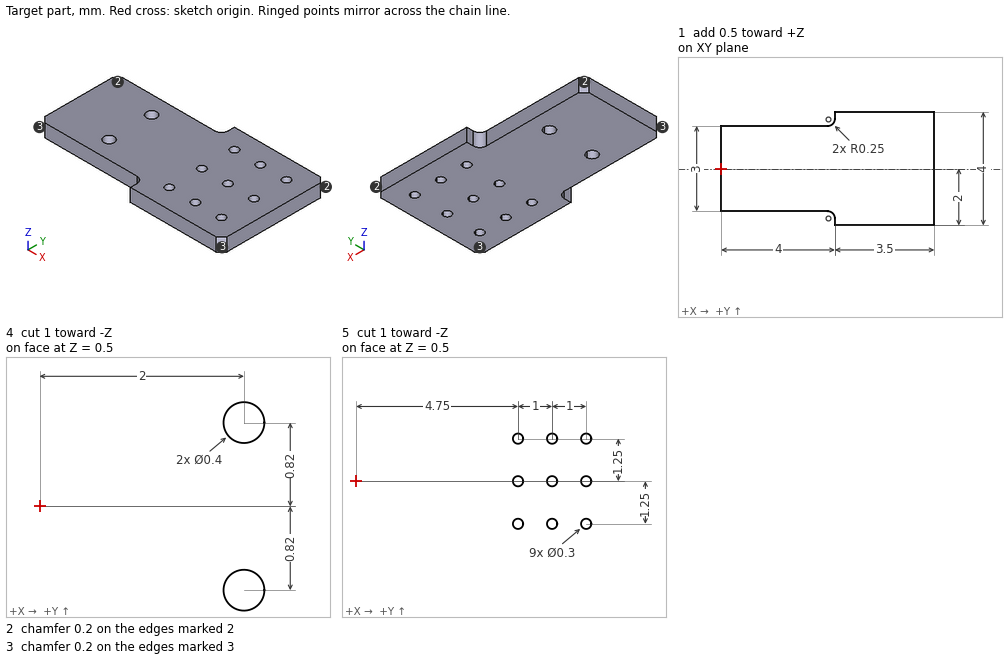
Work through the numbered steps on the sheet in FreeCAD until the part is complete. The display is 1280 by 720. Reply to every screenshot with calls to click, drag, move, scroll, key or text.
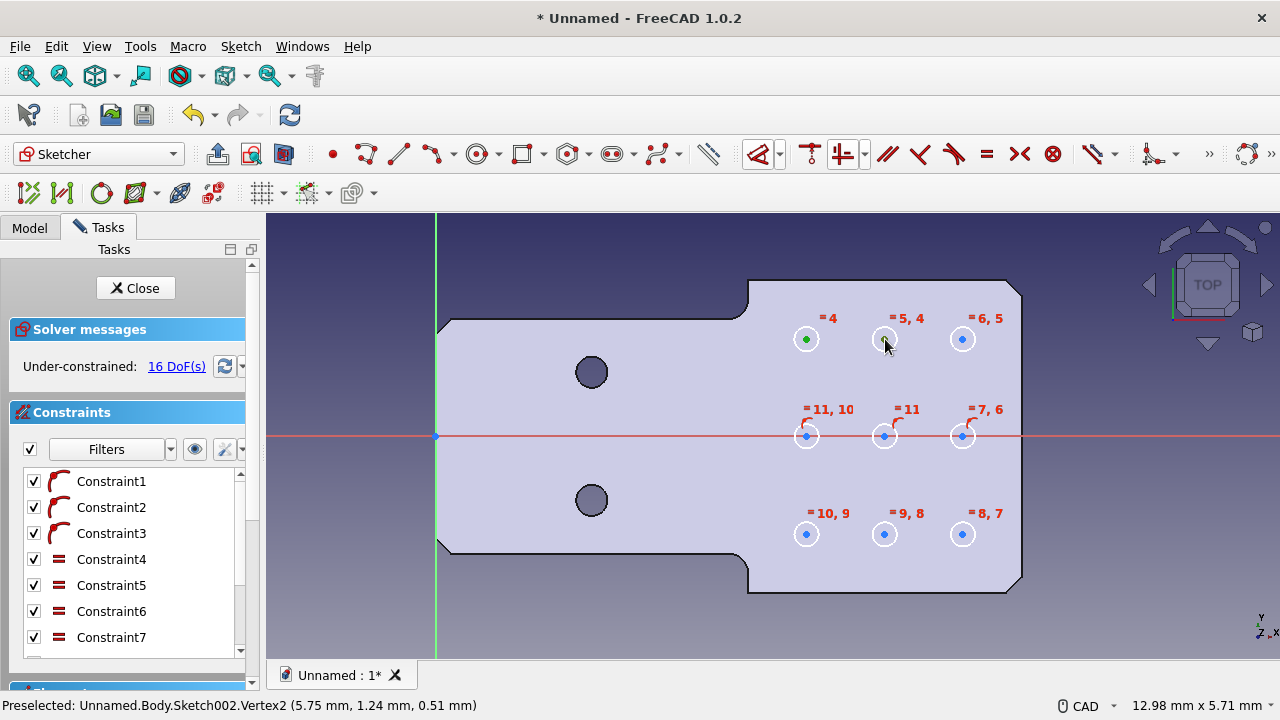
click(864, 154)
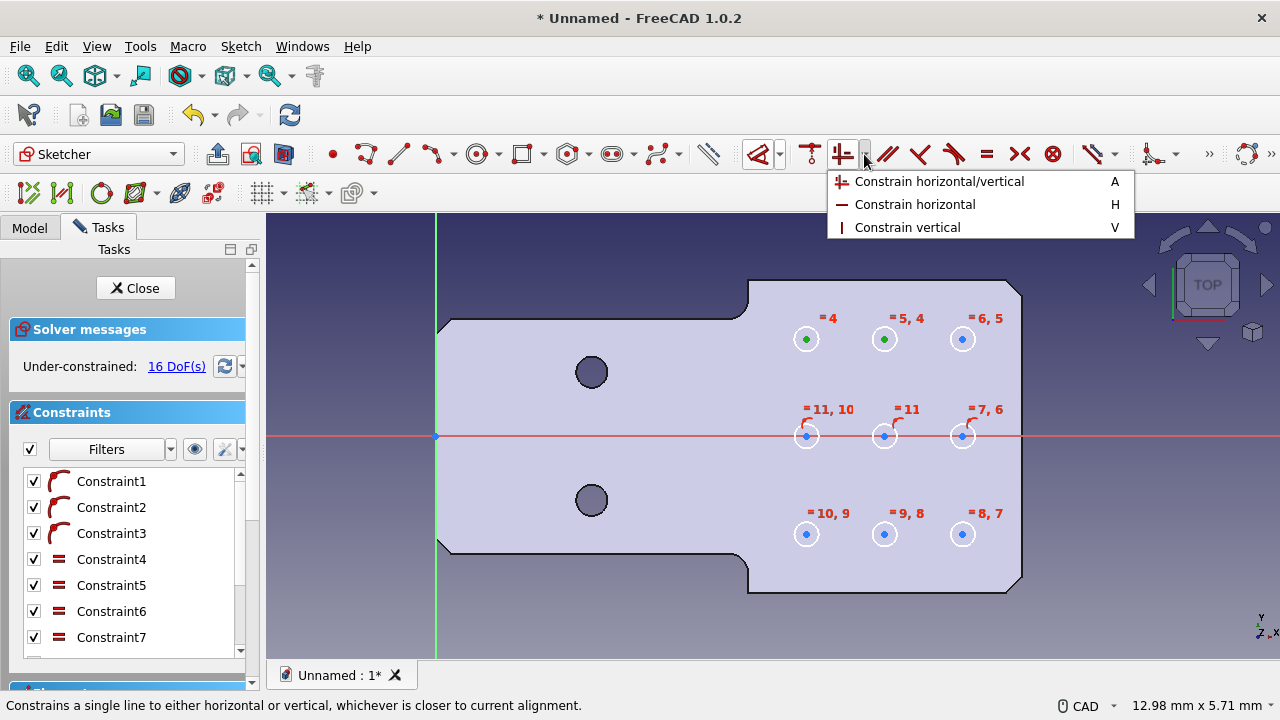
click(981, 204)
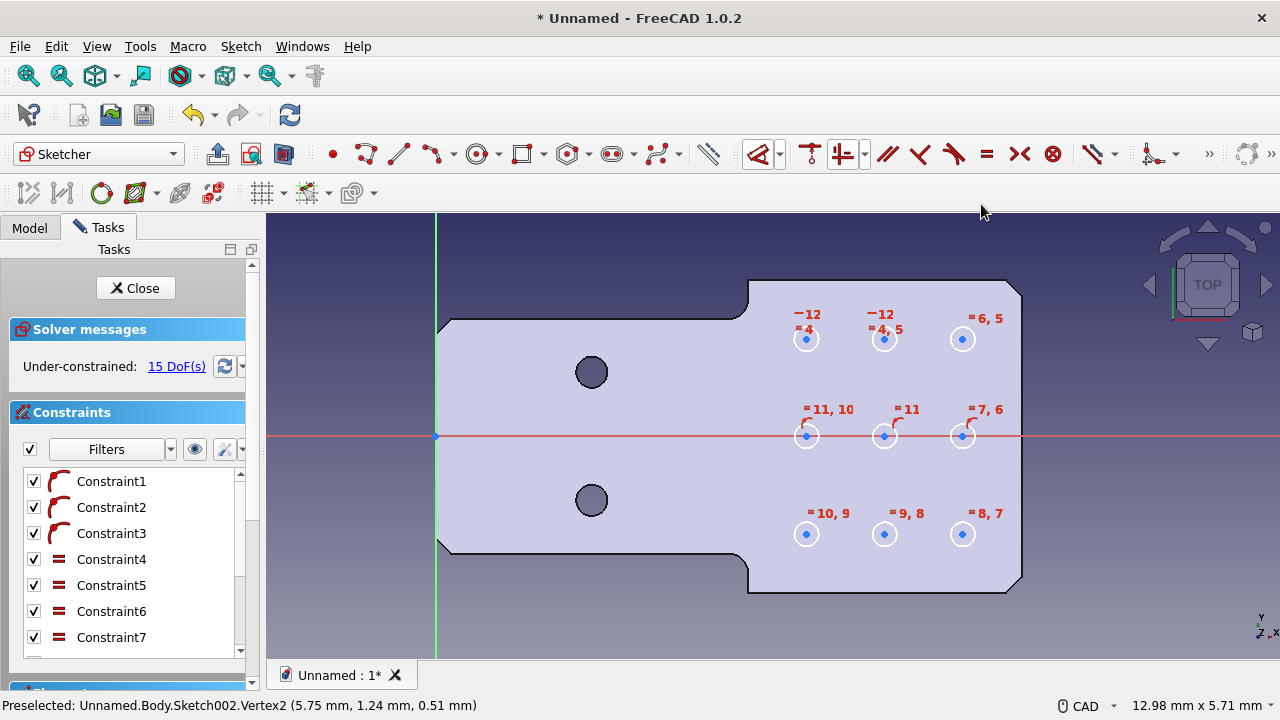
click(885, 339)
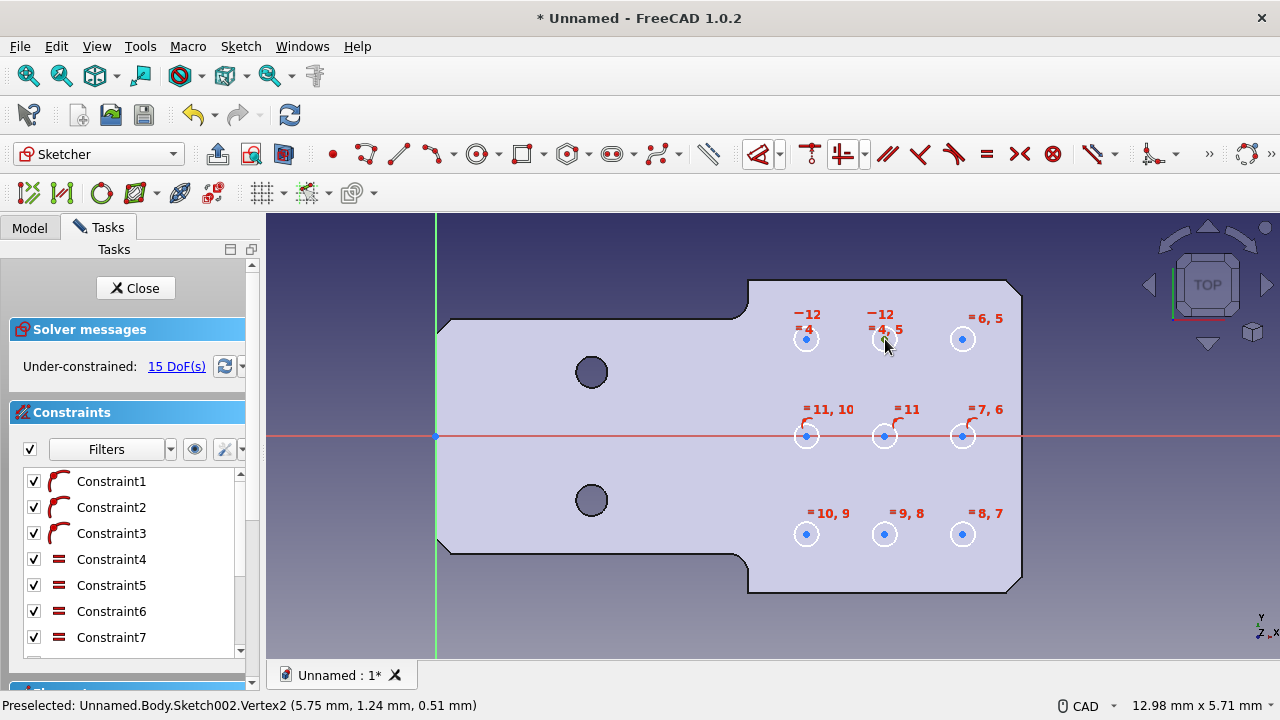
click(963, 339)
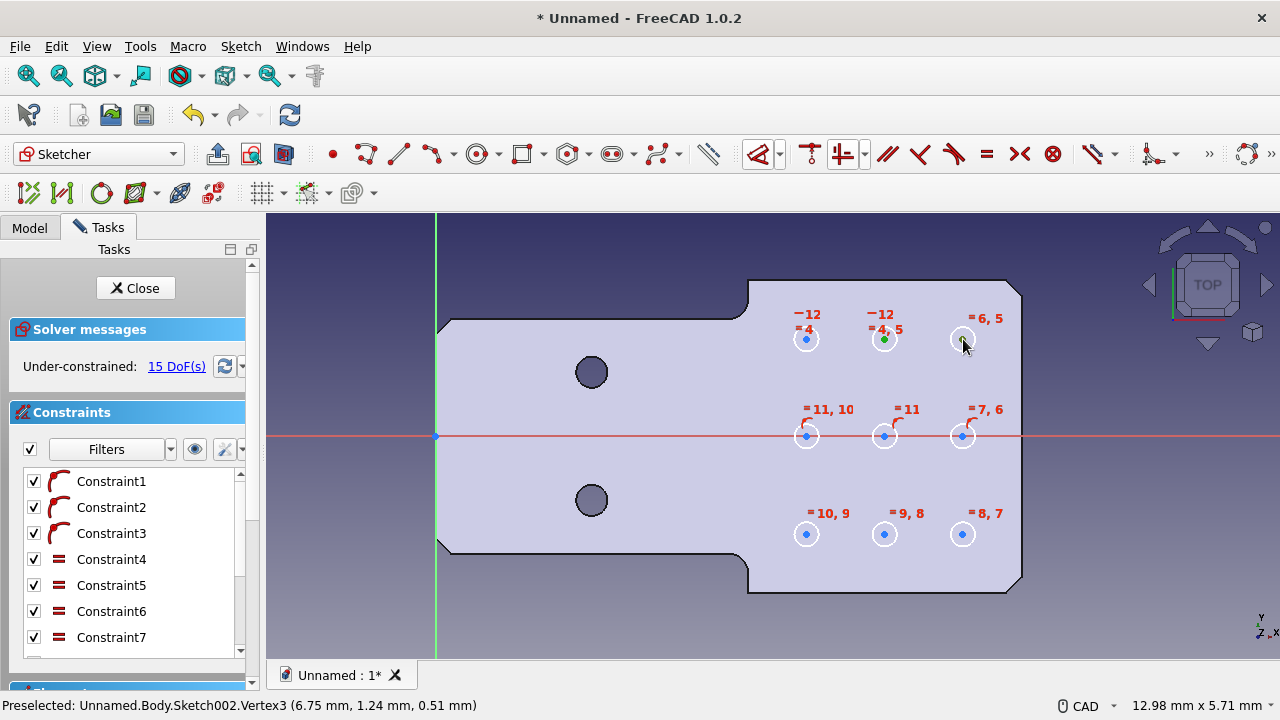
key(h)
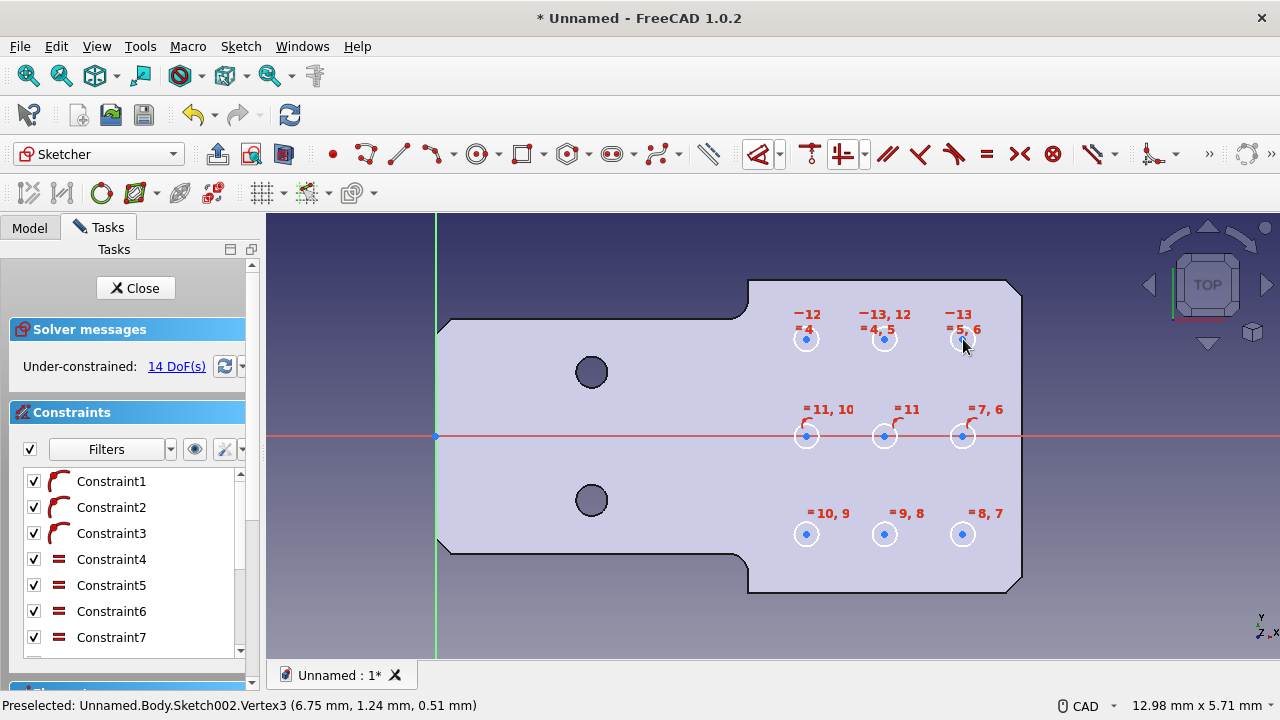
click(963, 339)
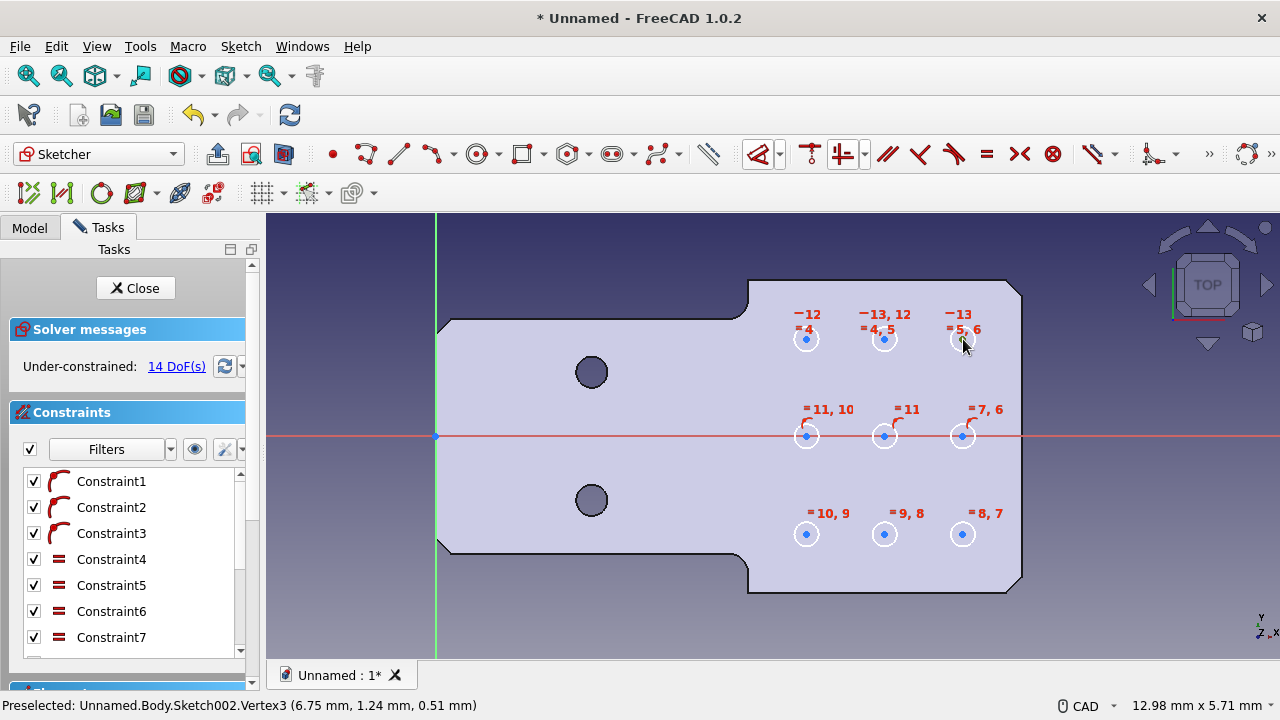
click(963, 436)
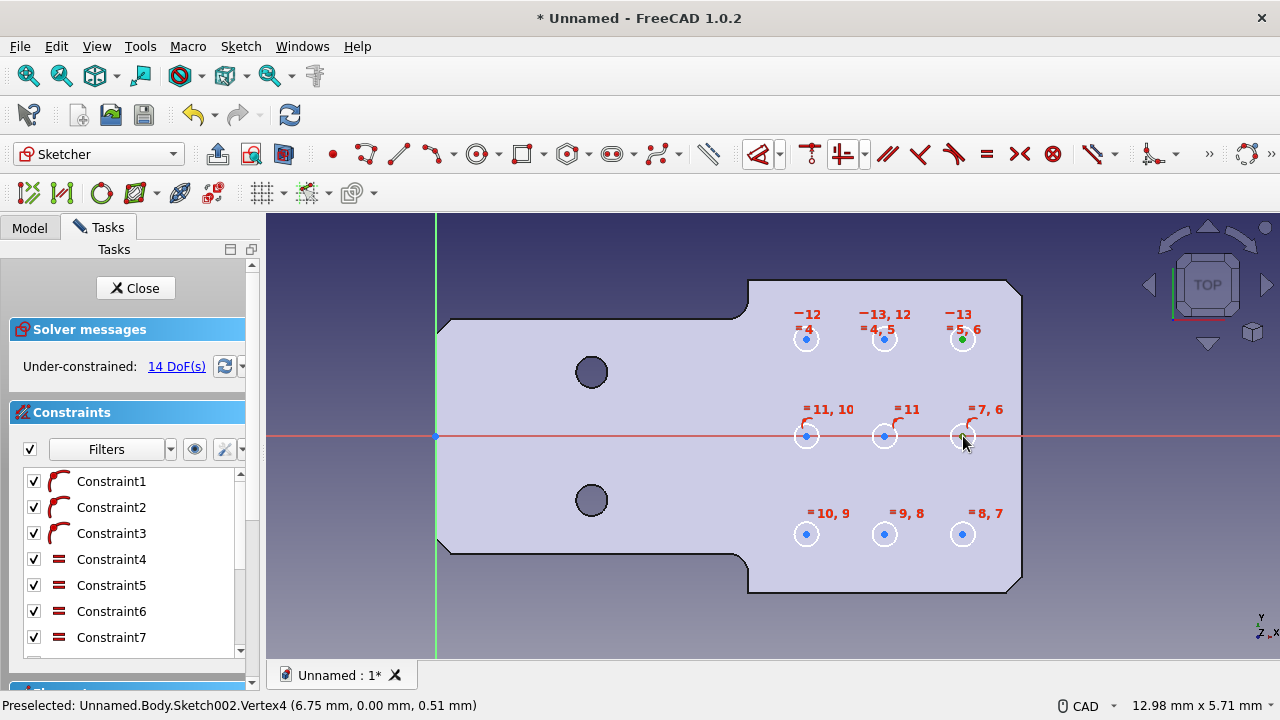
key(v)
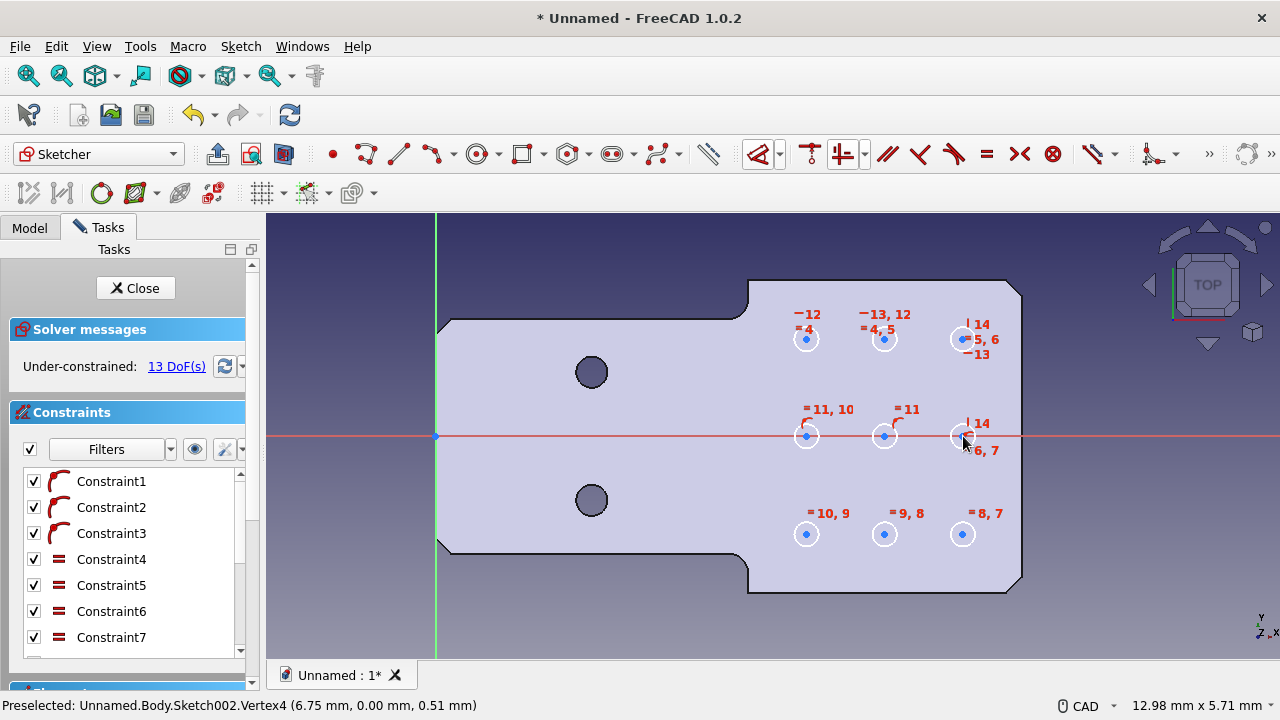
click(961, 438)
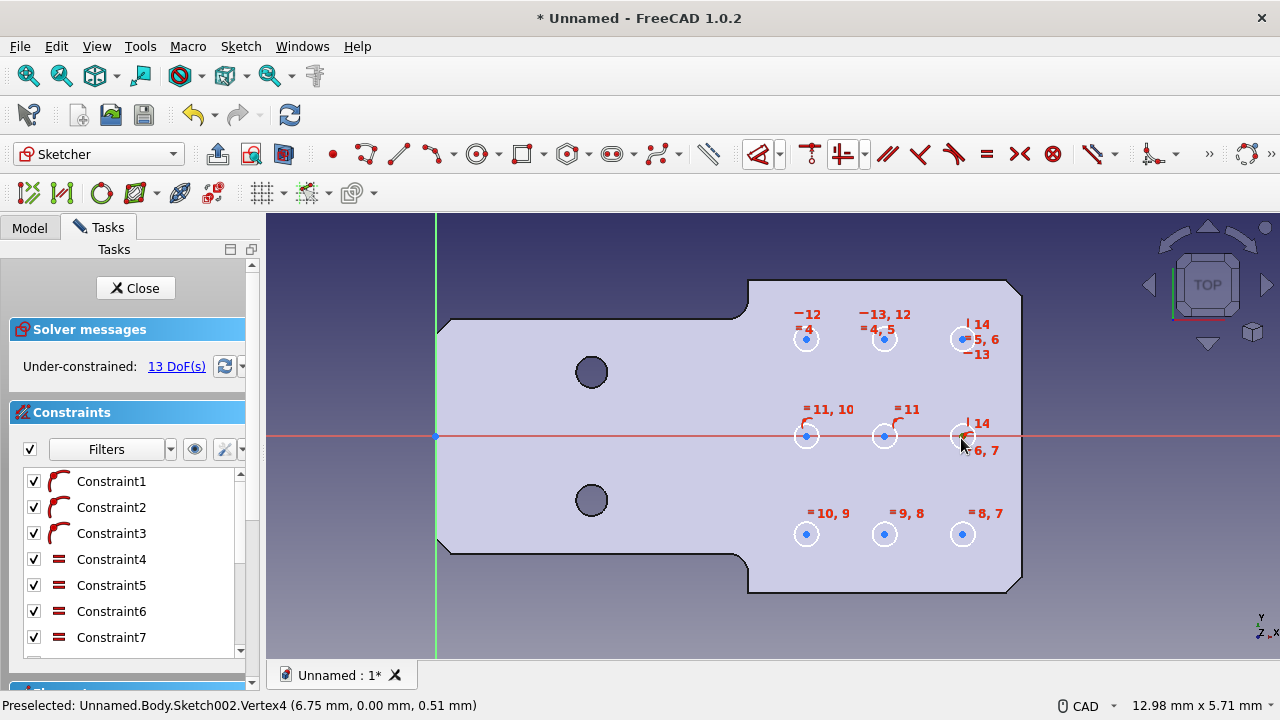
click(963, 534)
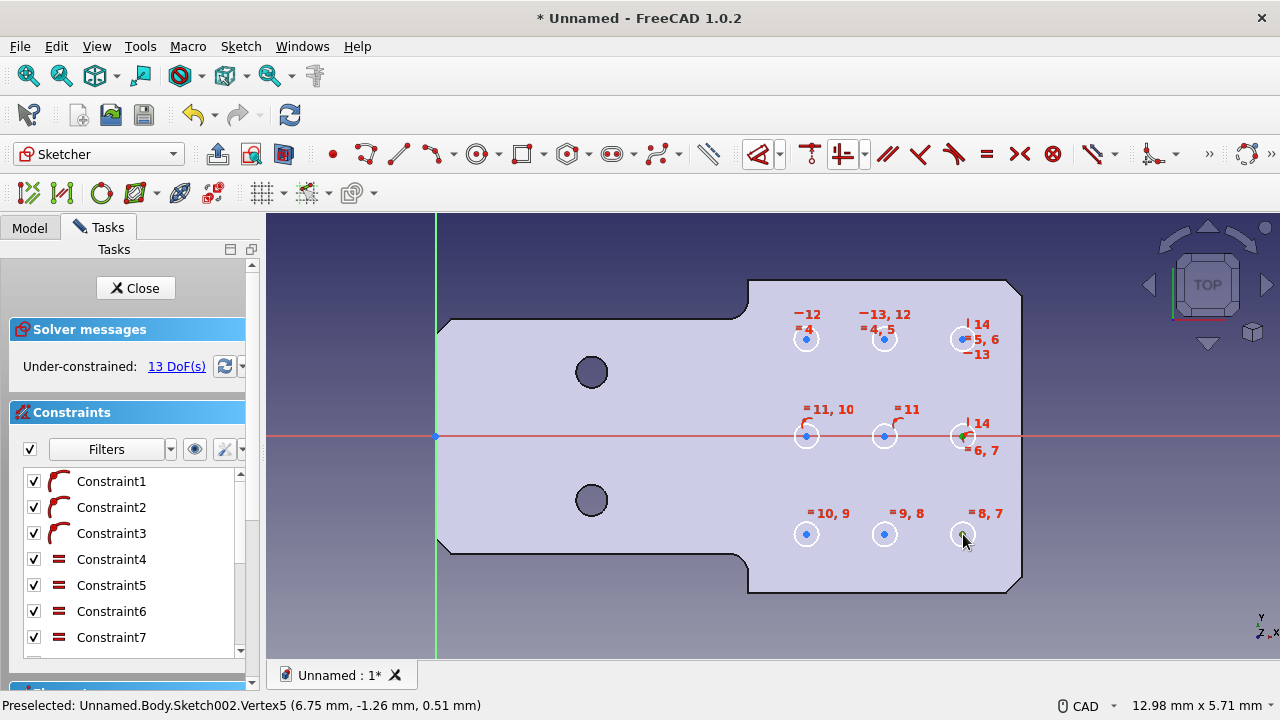
key(v)